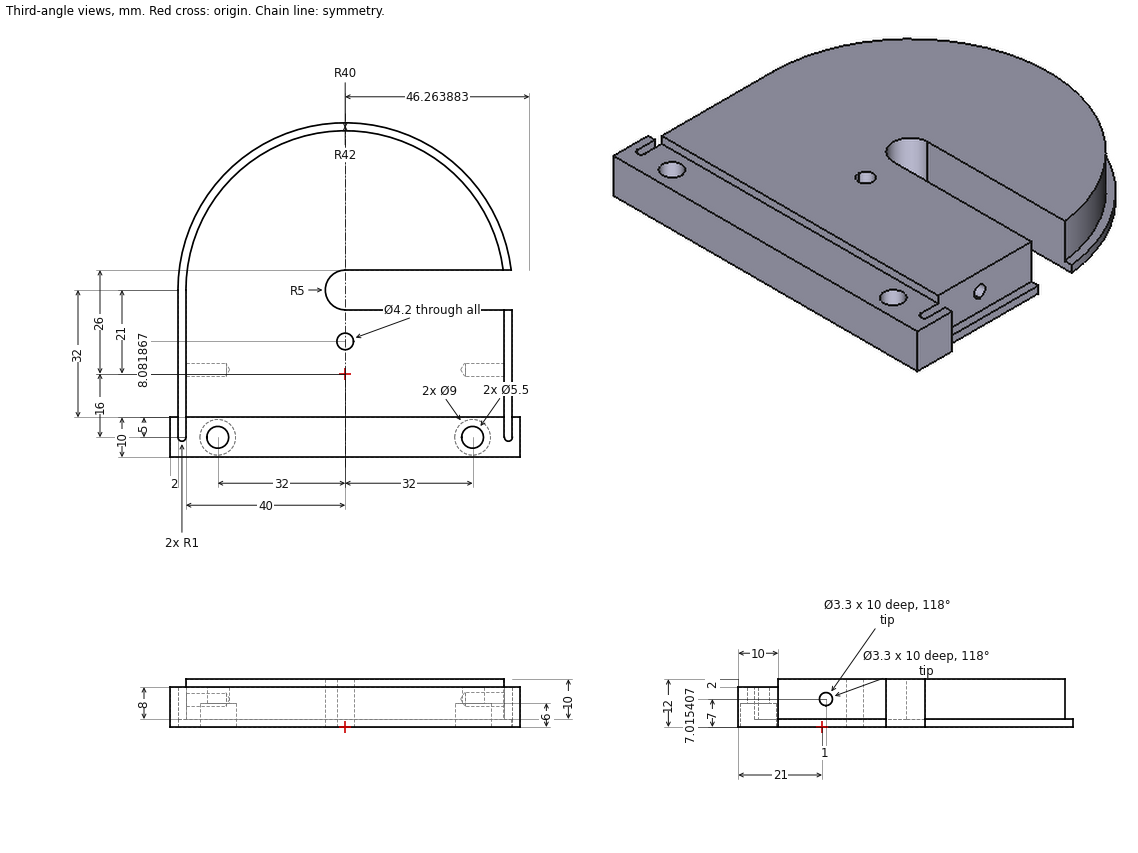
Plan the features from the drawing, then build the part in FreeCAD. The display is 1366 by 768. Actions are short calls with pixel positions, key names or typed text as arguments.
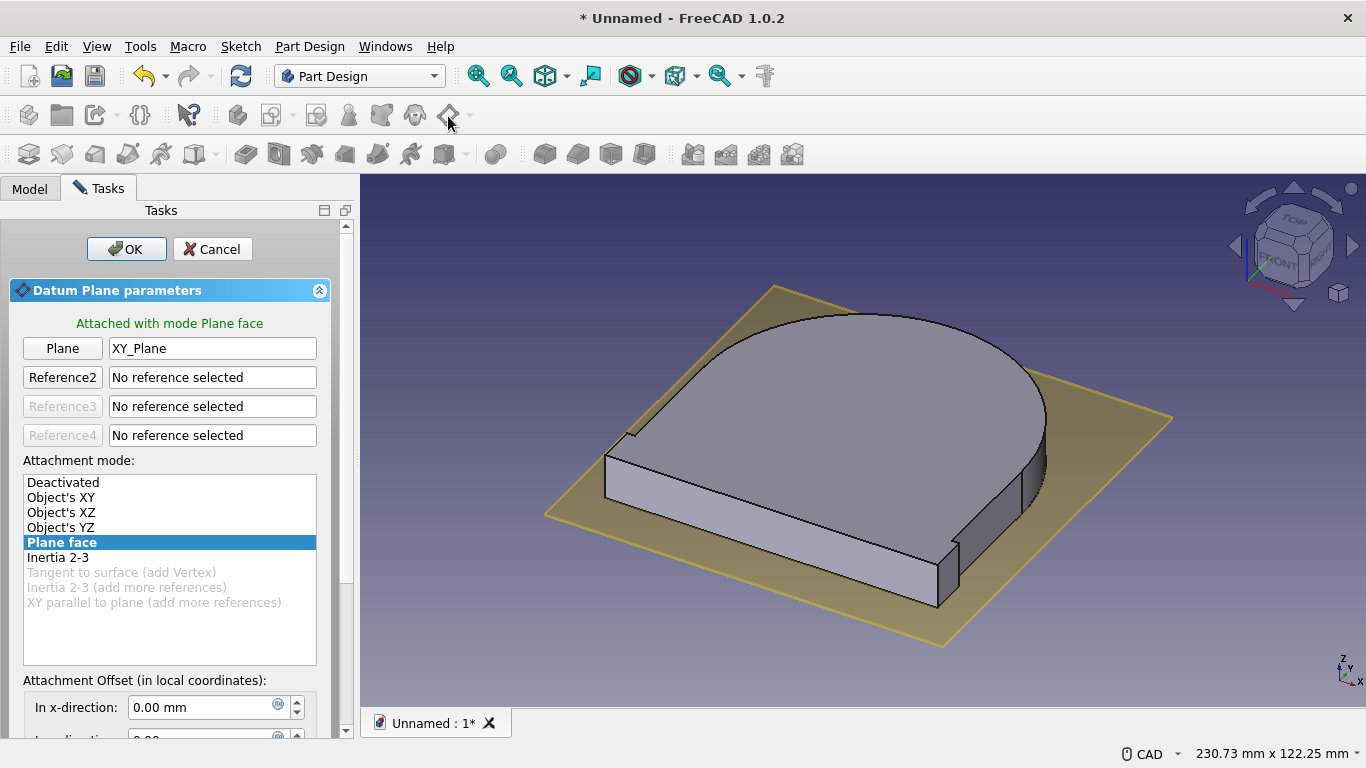
scroll(346, 479, down, 2)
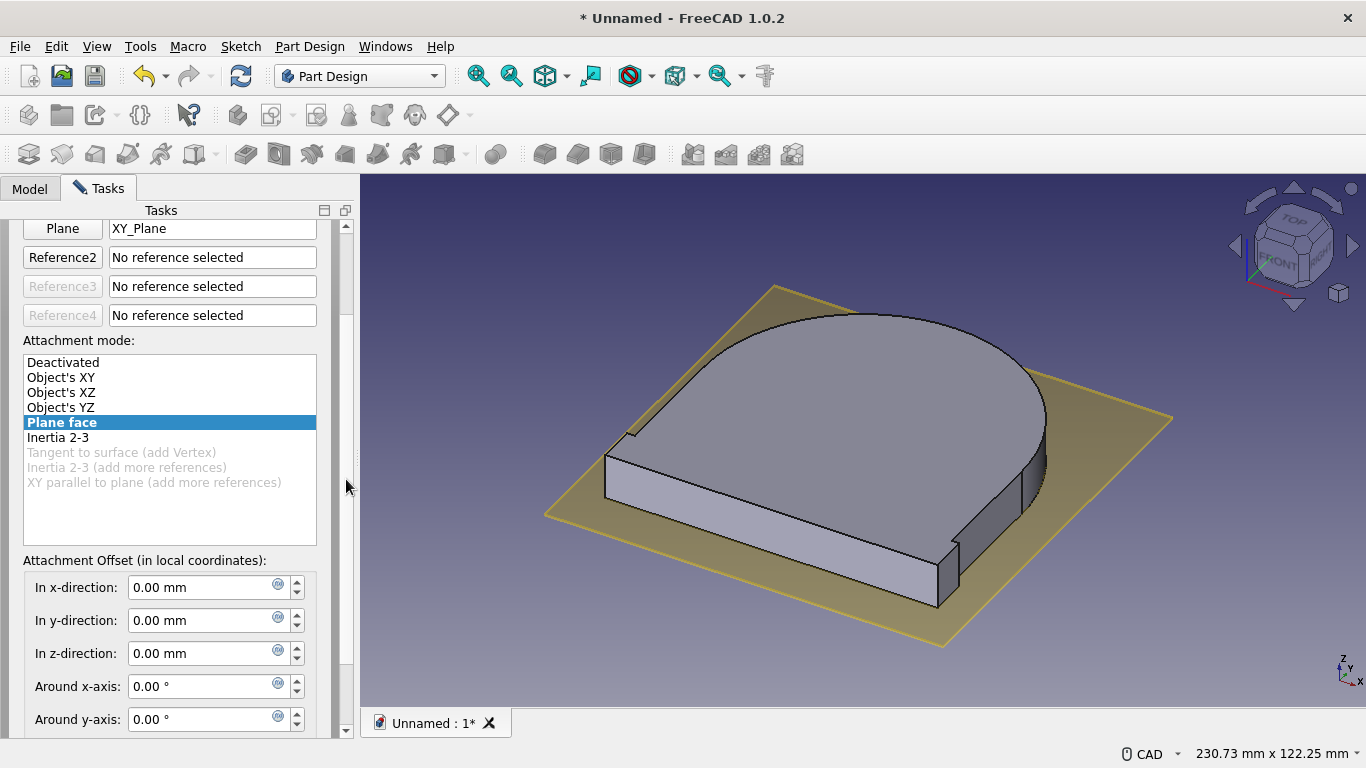
triple_click(210, 654)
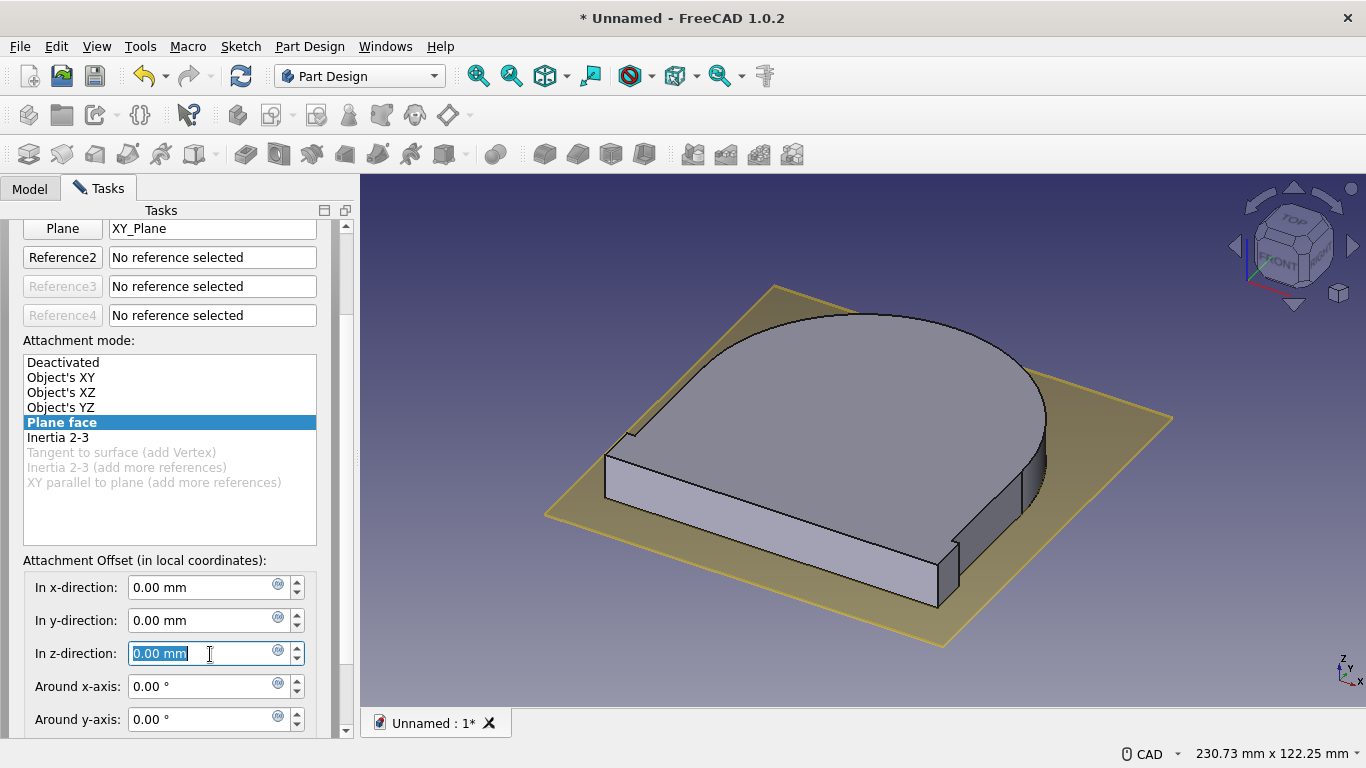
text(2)
key(Tab)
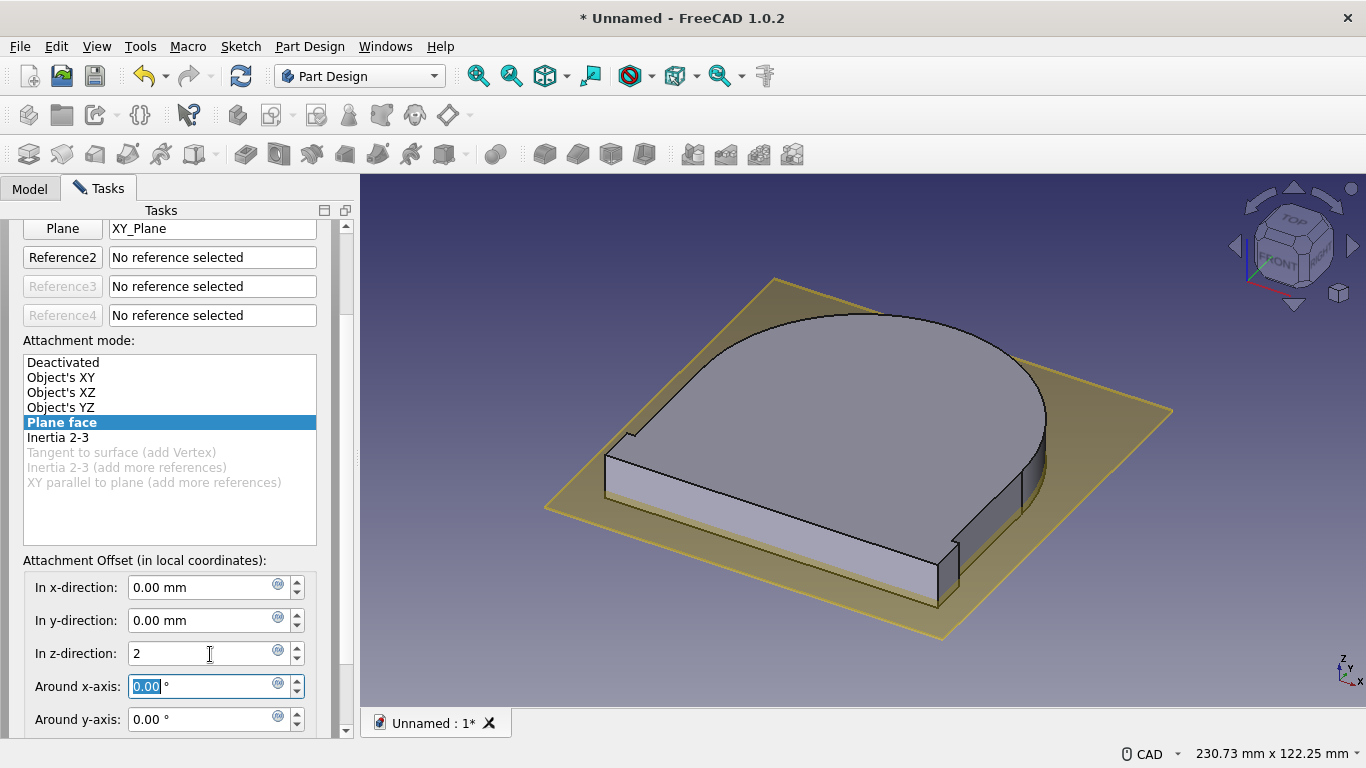
scroll(346, 479, up, 3)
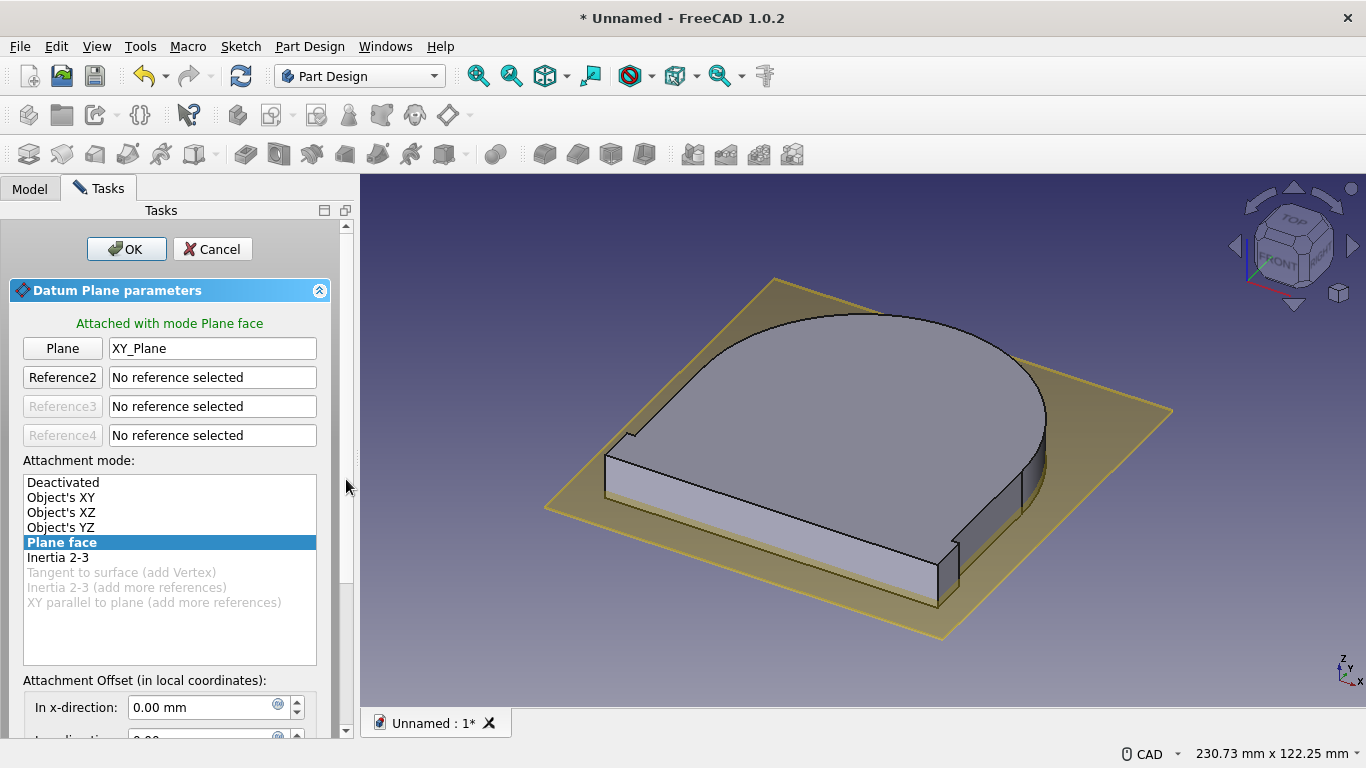
click(127, 249)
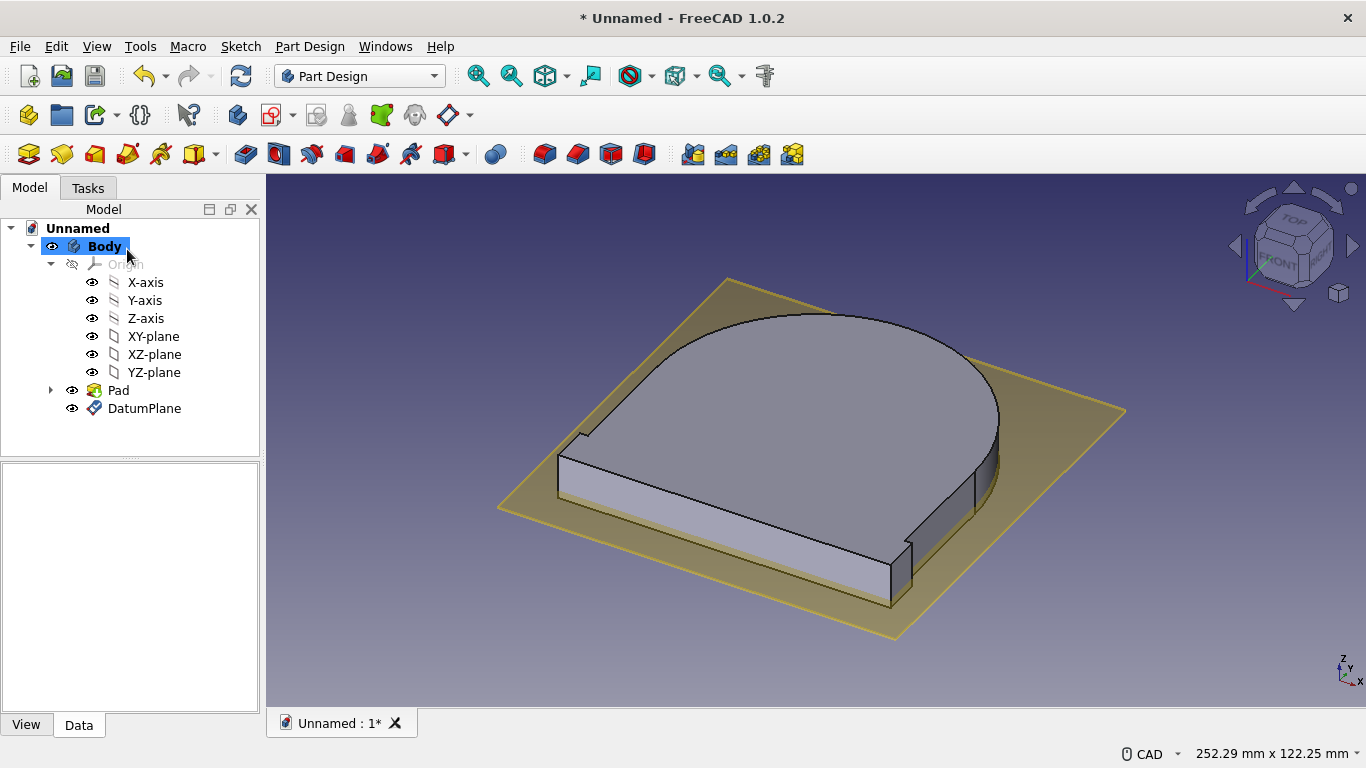
click(117, 408)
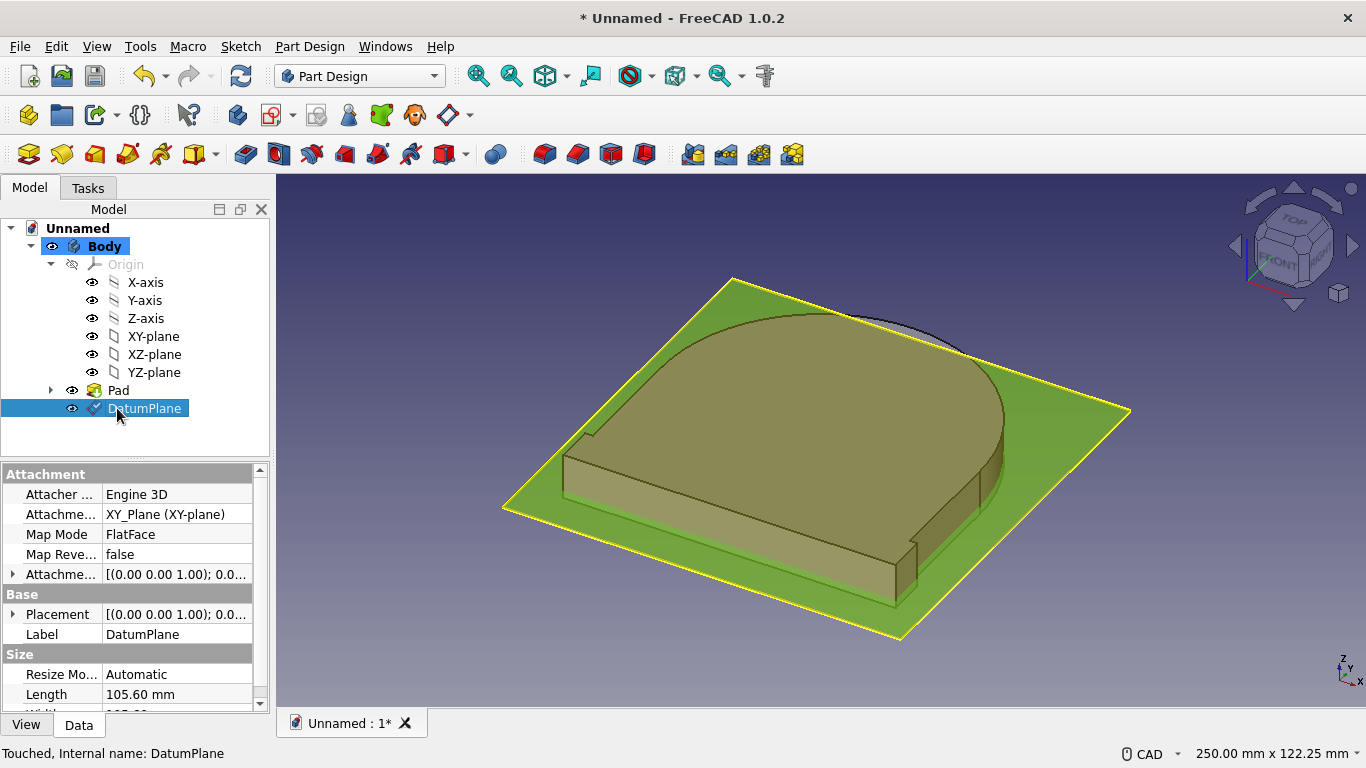
click(270, 116)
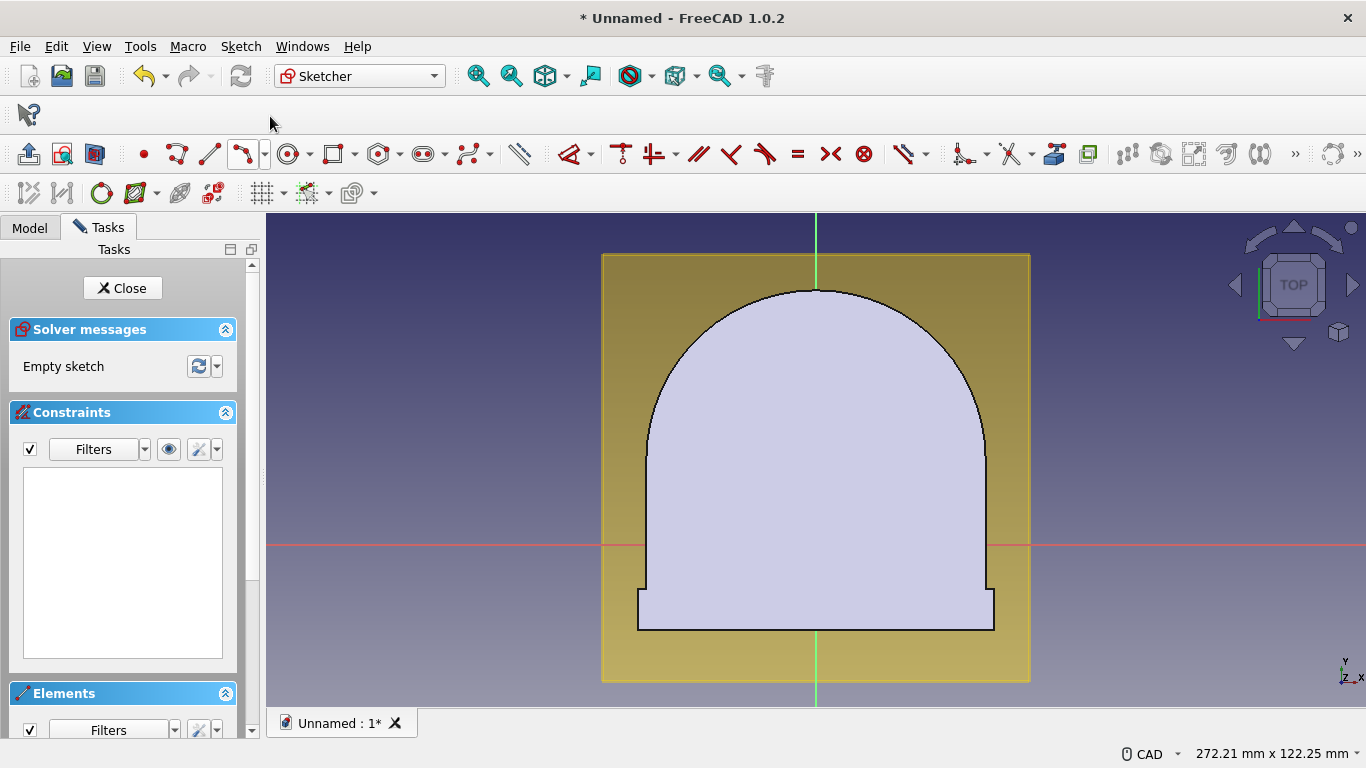
click(95, 154)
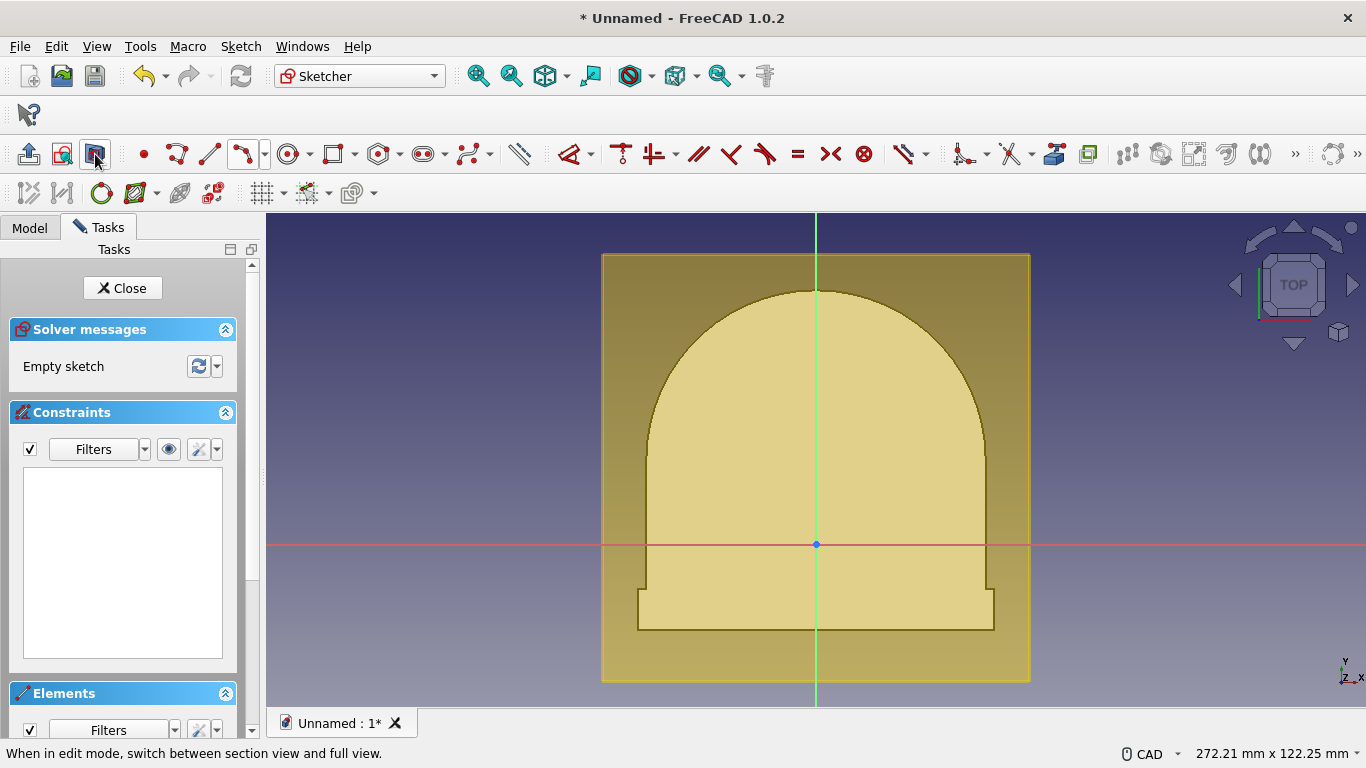
click(177, 154)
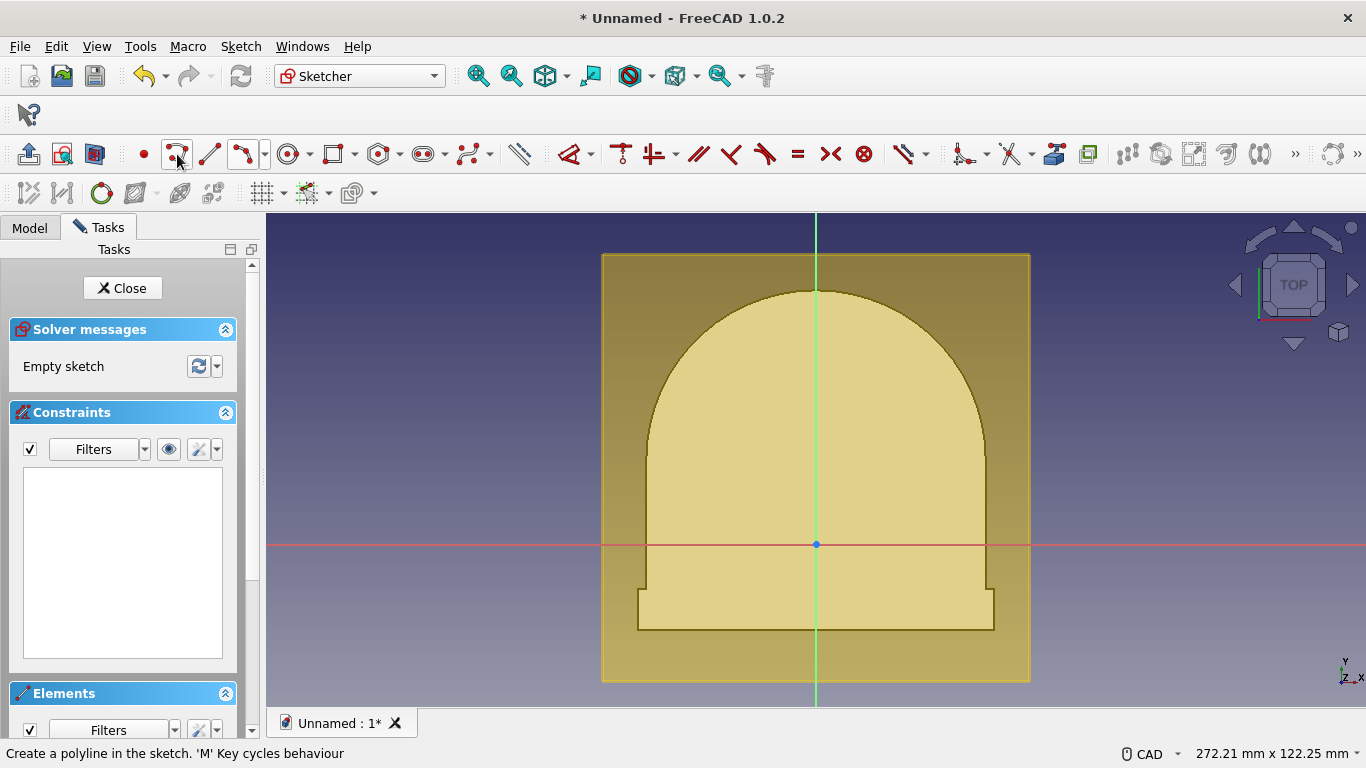
click(978, 460)
click(978, 589)